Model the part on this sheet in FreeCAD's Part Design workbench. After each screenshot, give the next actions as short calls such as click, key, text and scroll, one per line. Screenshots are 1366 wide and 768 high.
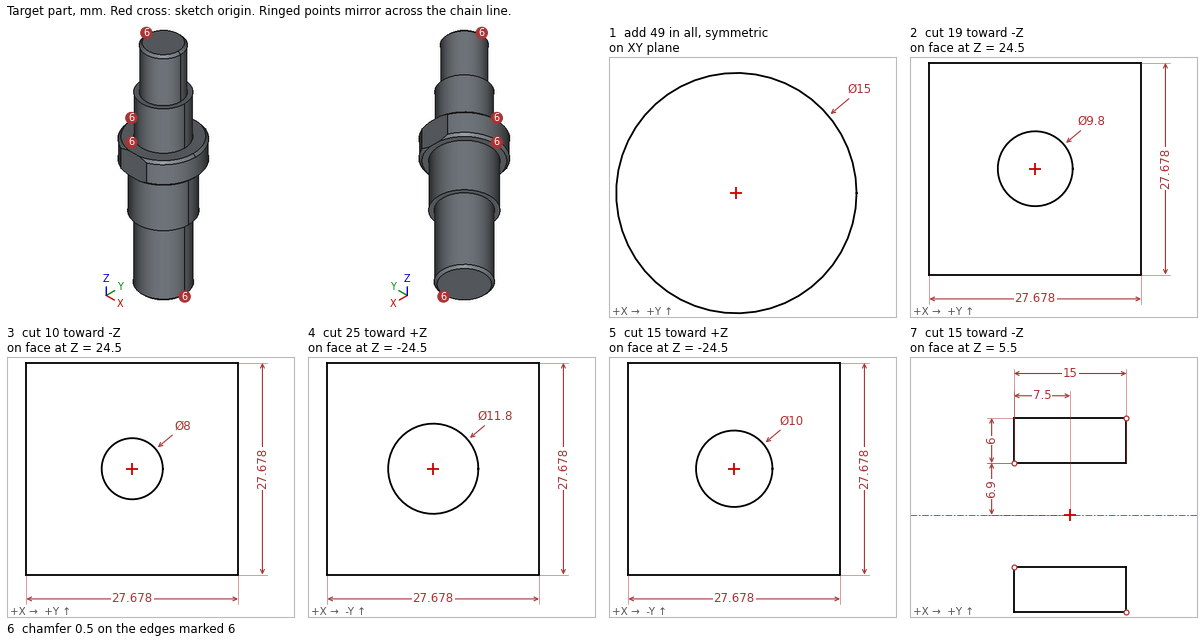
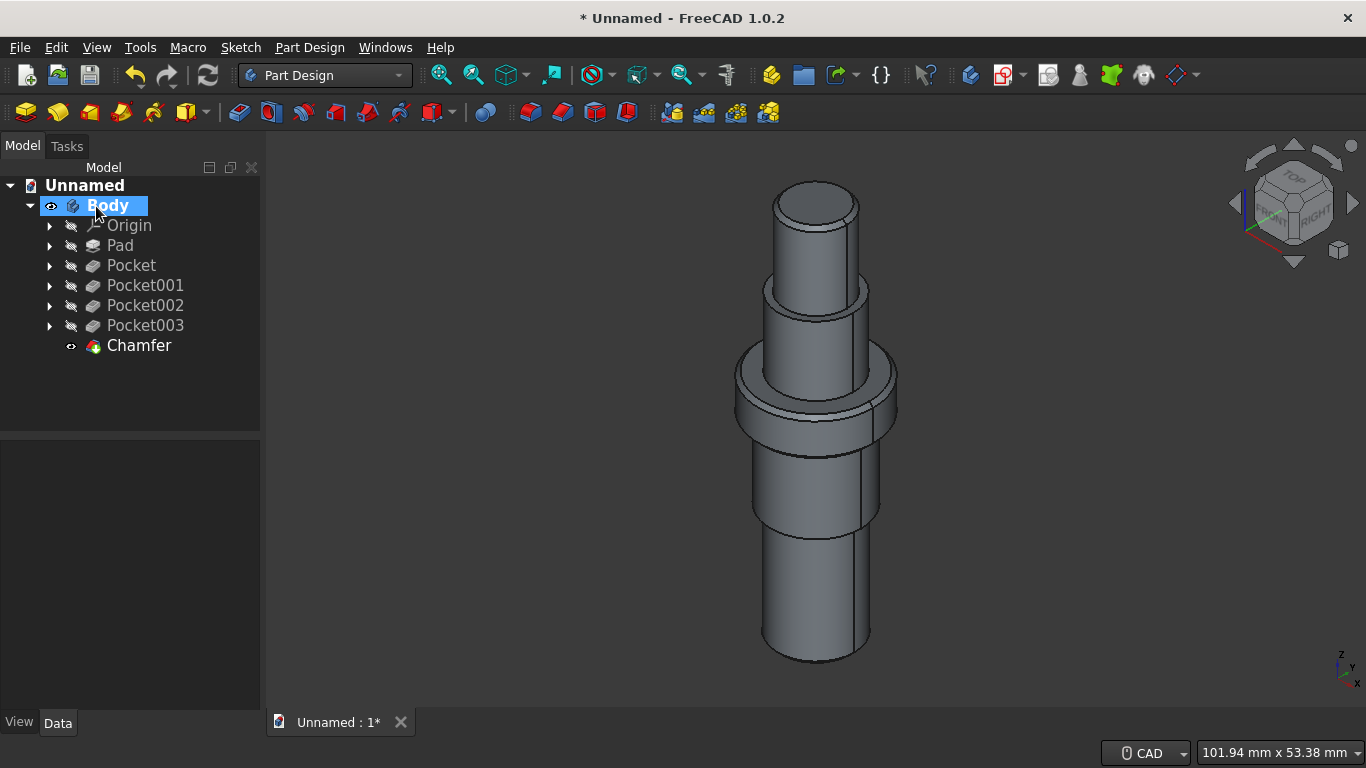
click(877, 370)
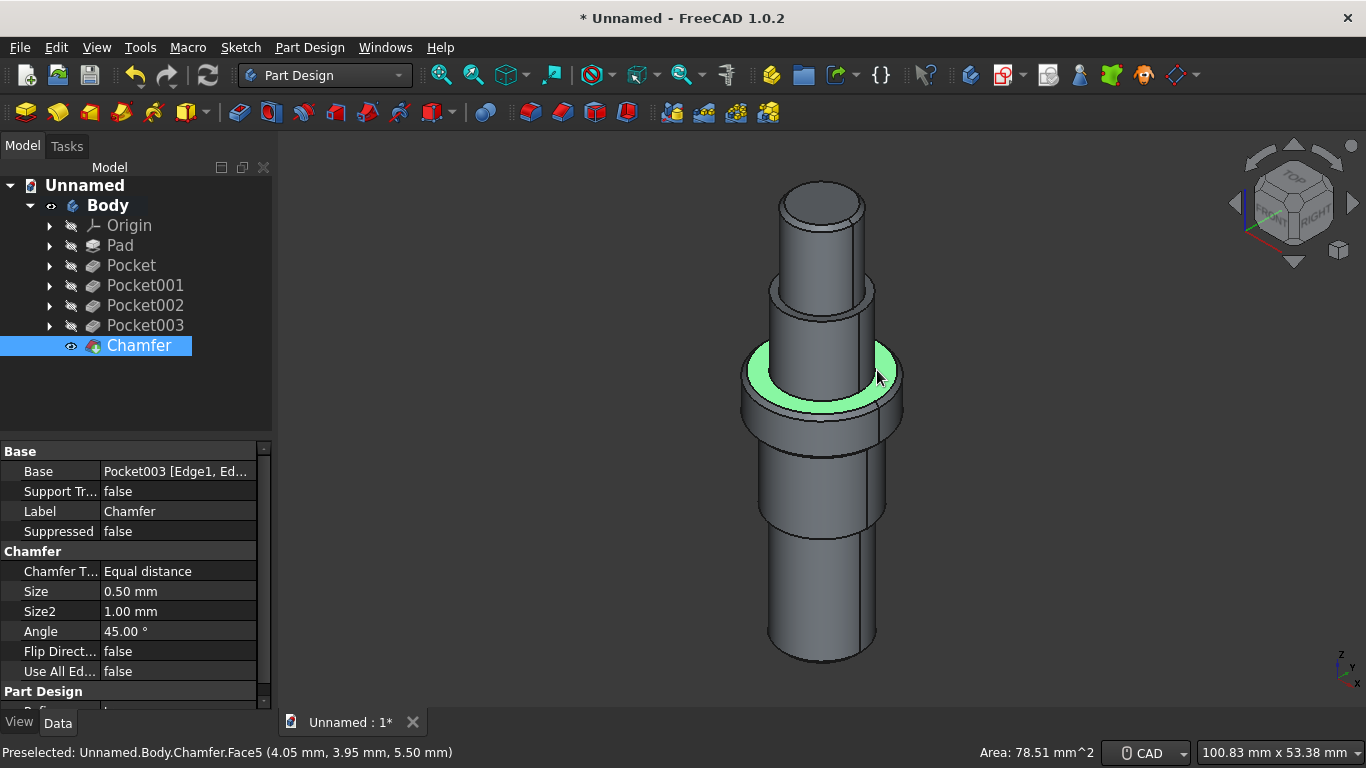
click(1004, 76)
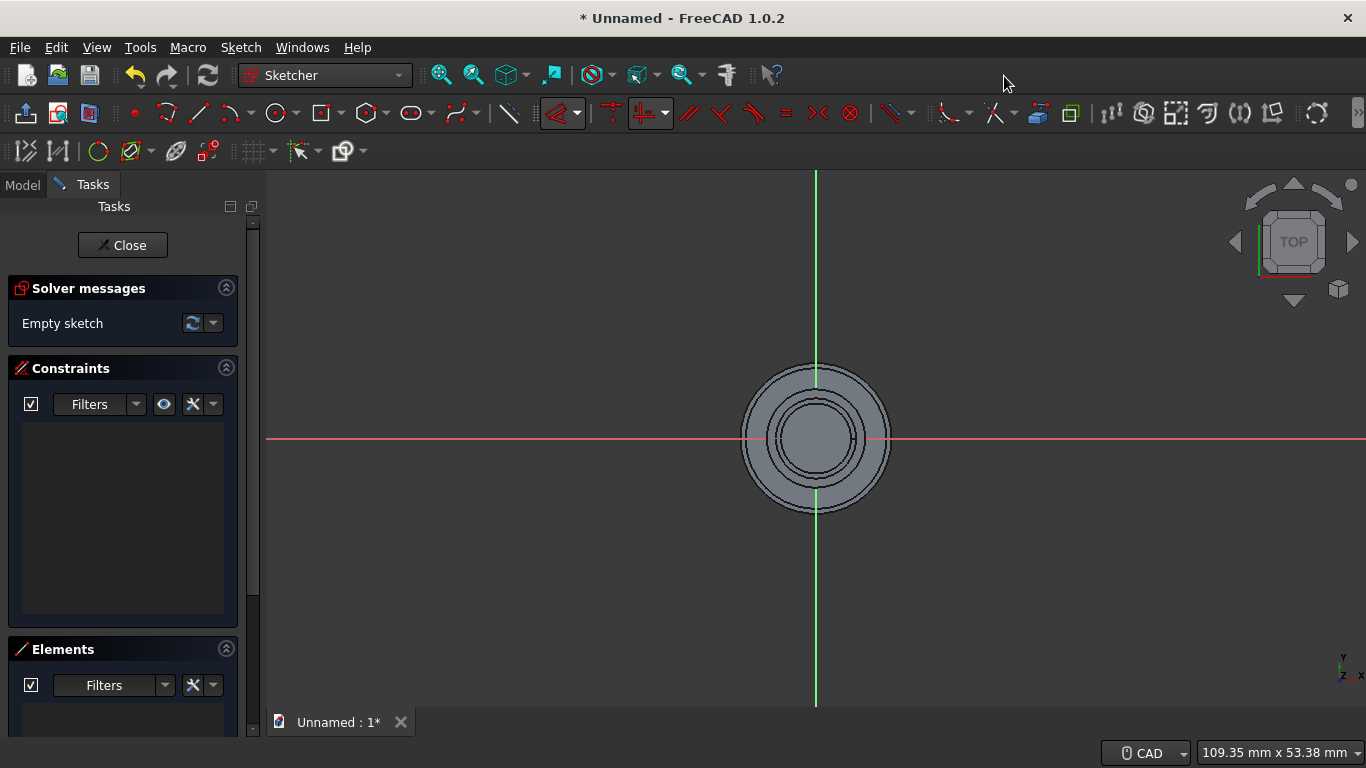
click(90, 114)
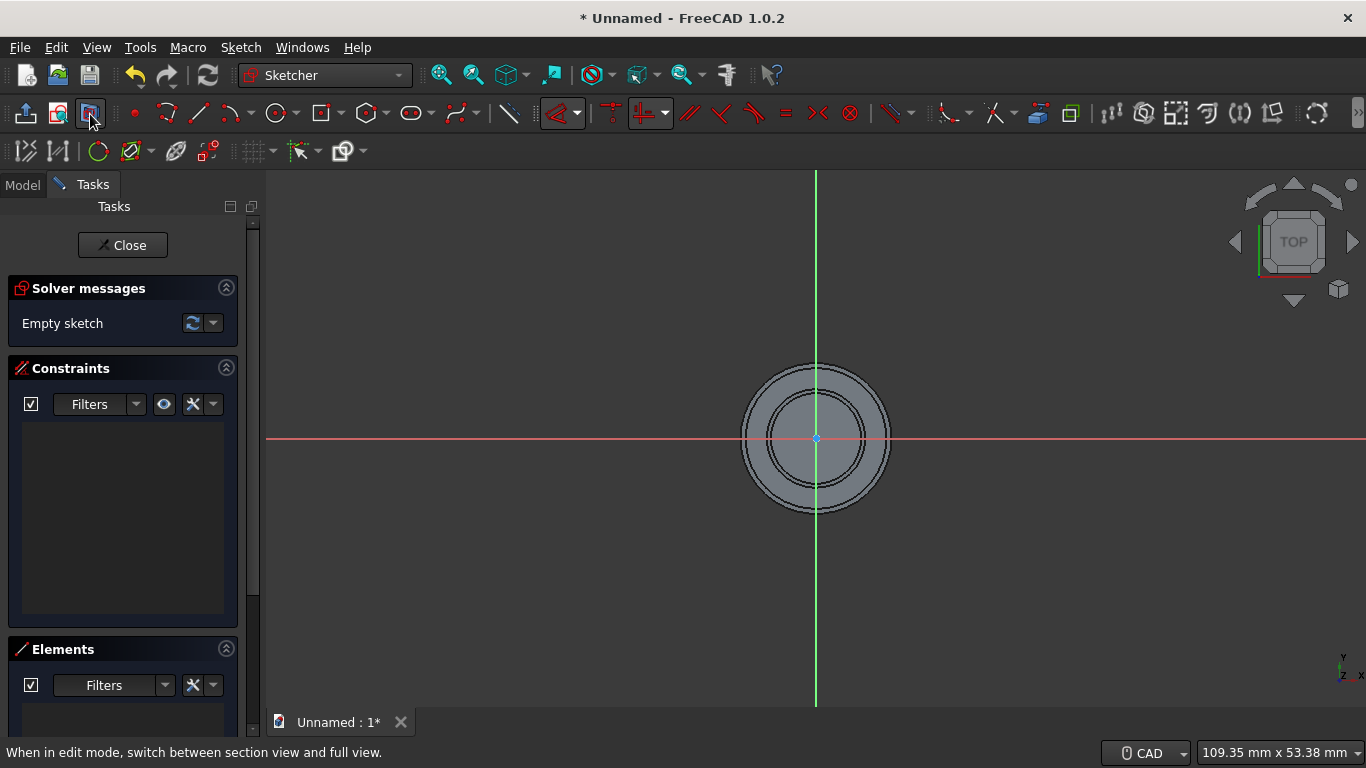
key(g)
key(r)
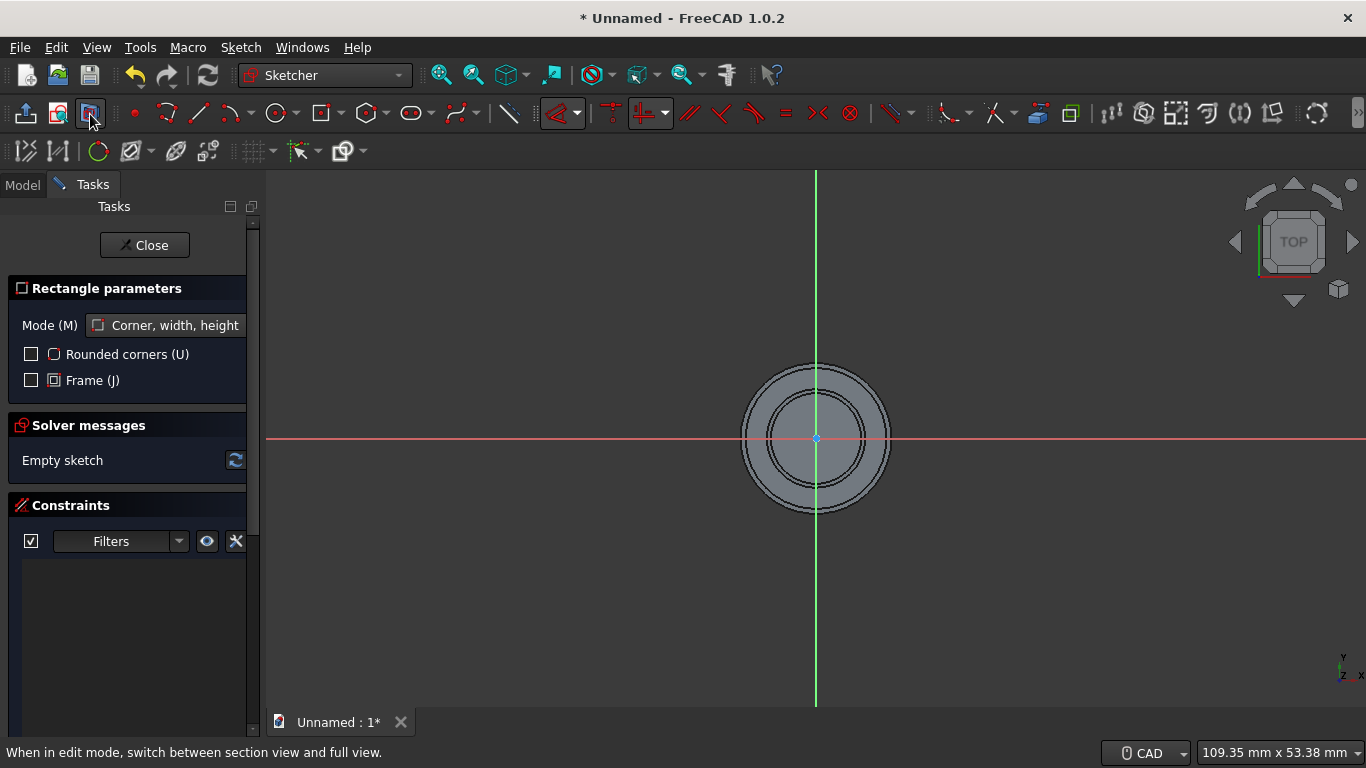
click(741, 309)
click(891, 369)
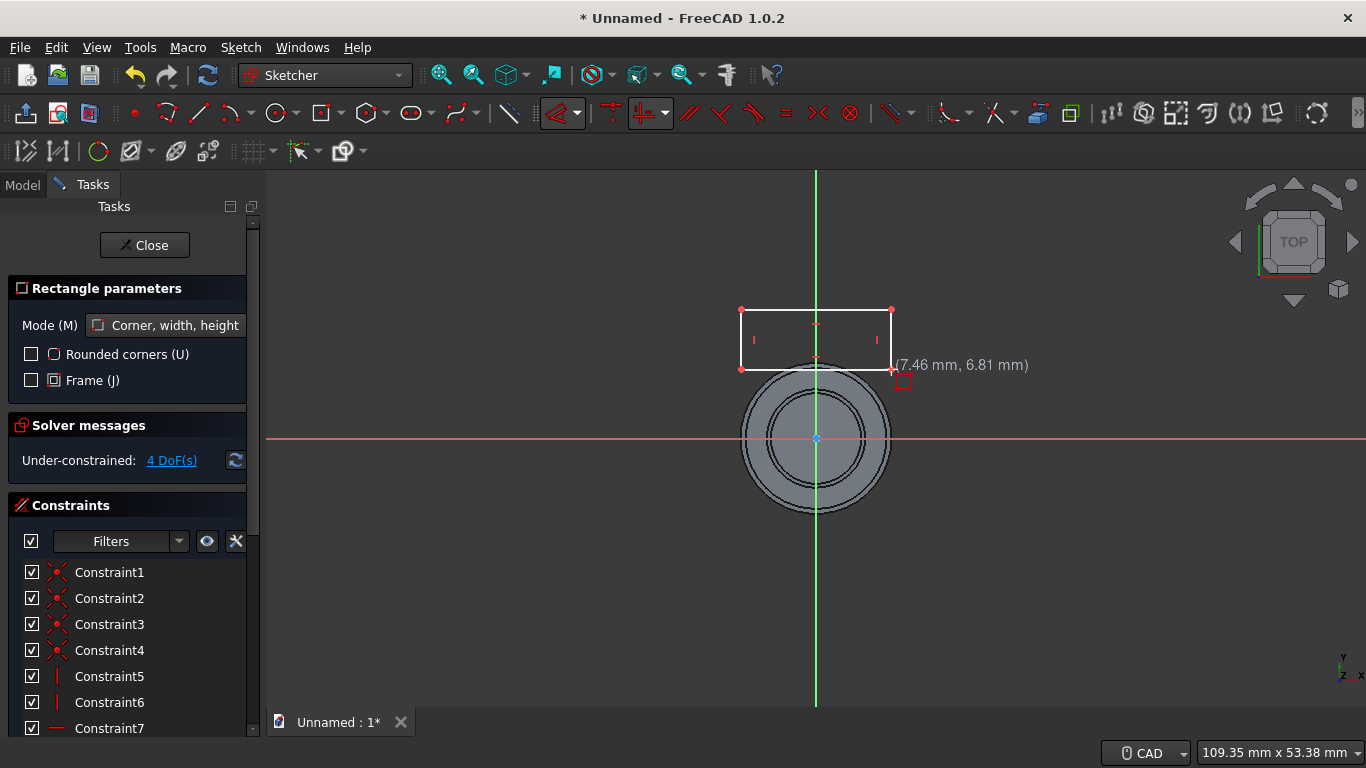
click(741, 508)
click(891, 568)
key(Escape)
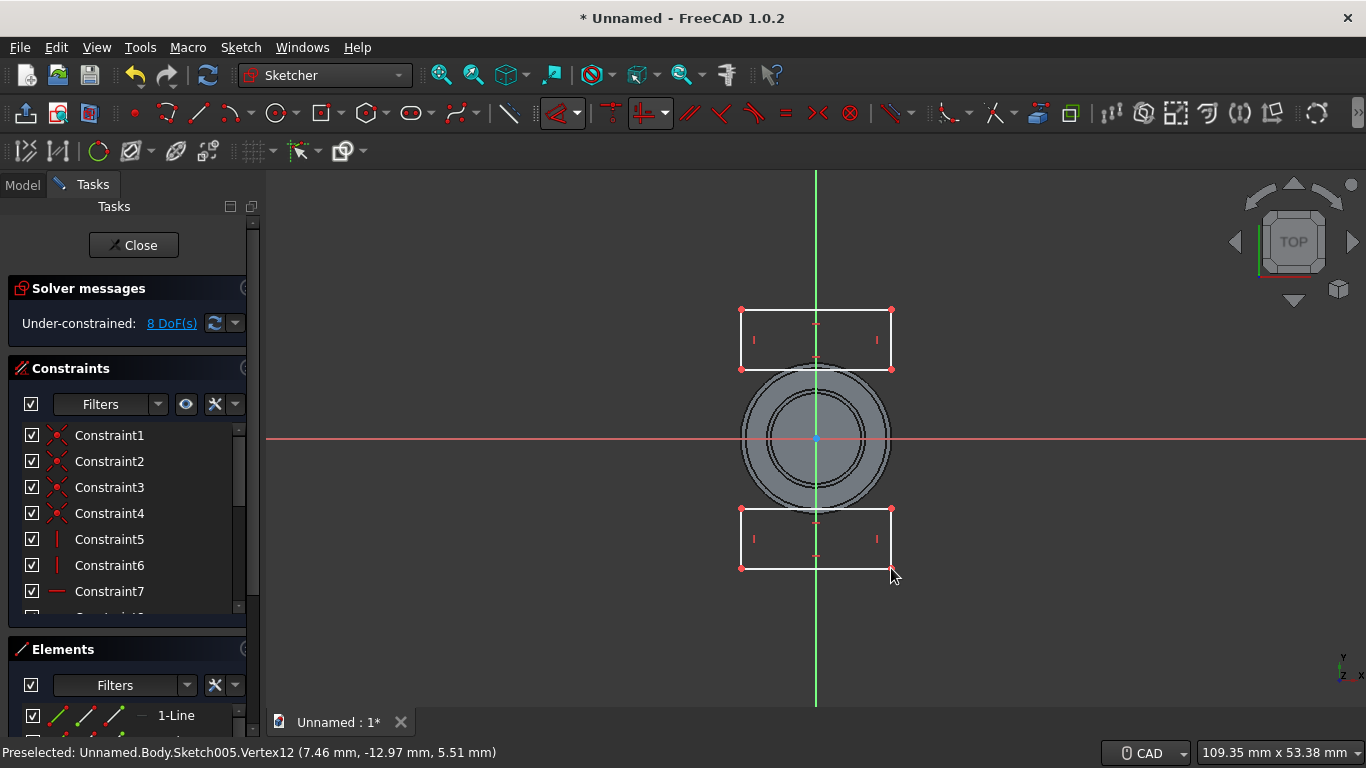
click(741, 370)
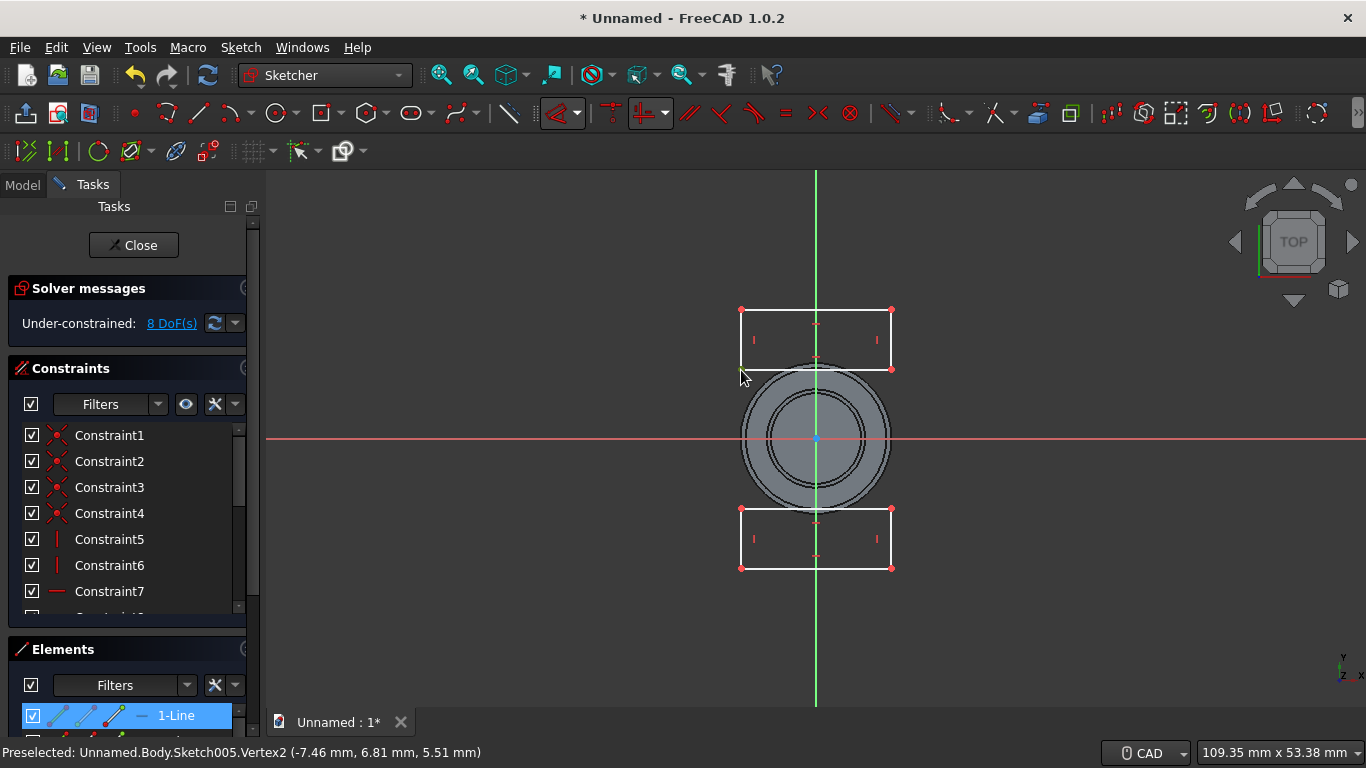
click(741, 509)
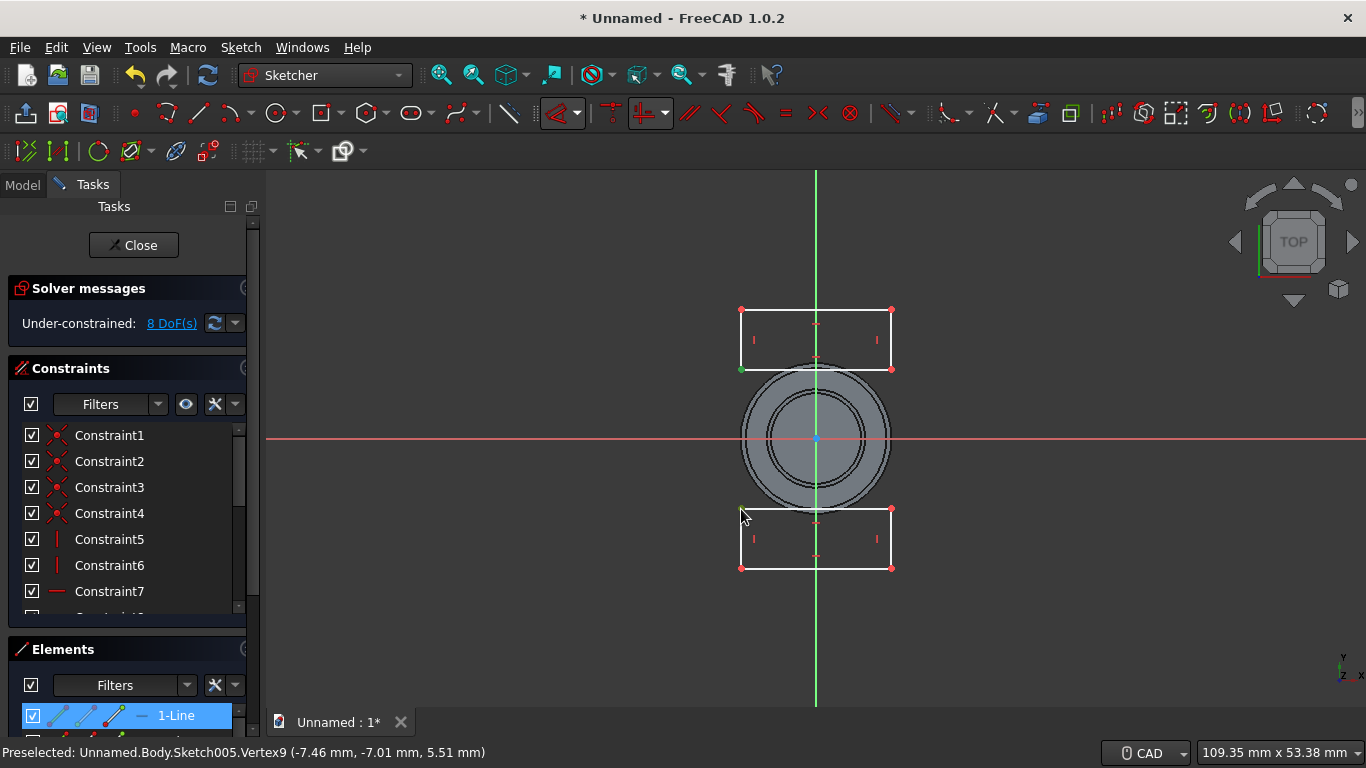
click(359, 439)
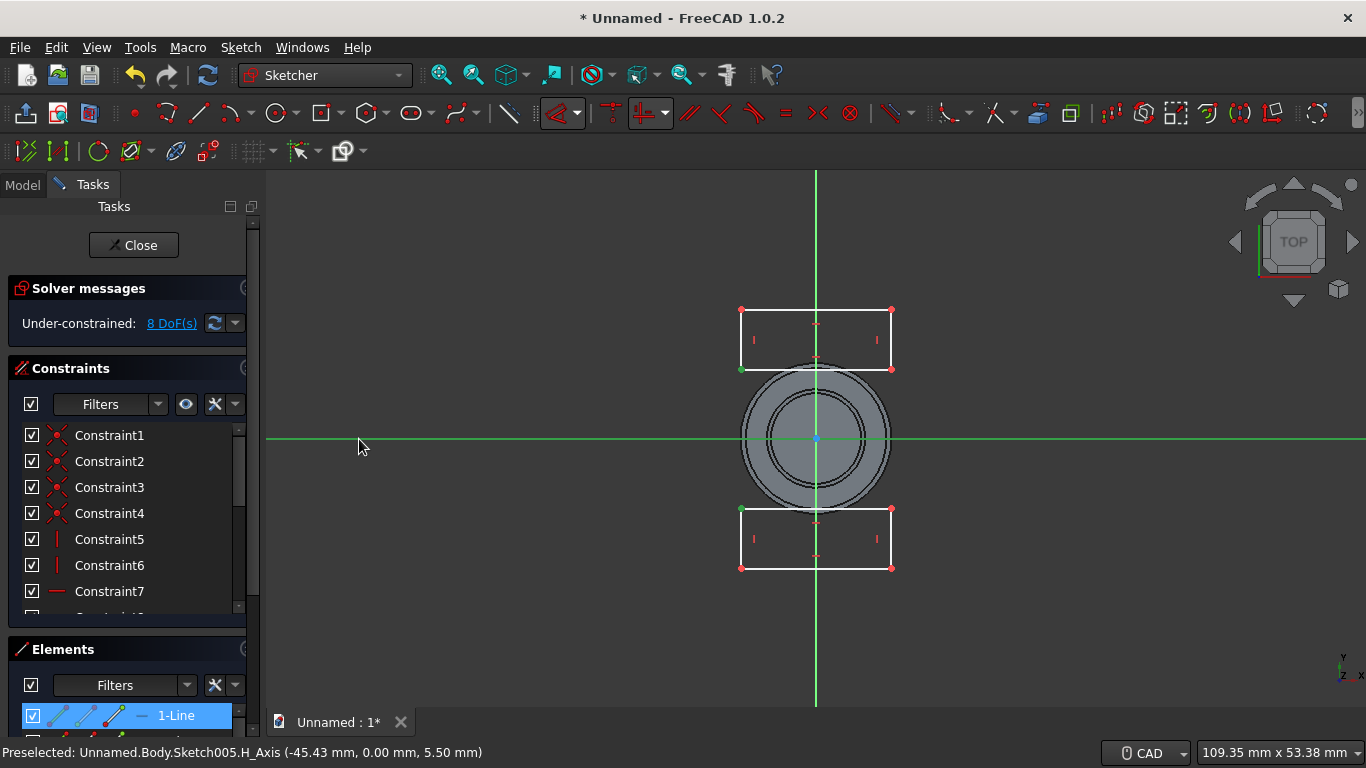
click(818, 114)